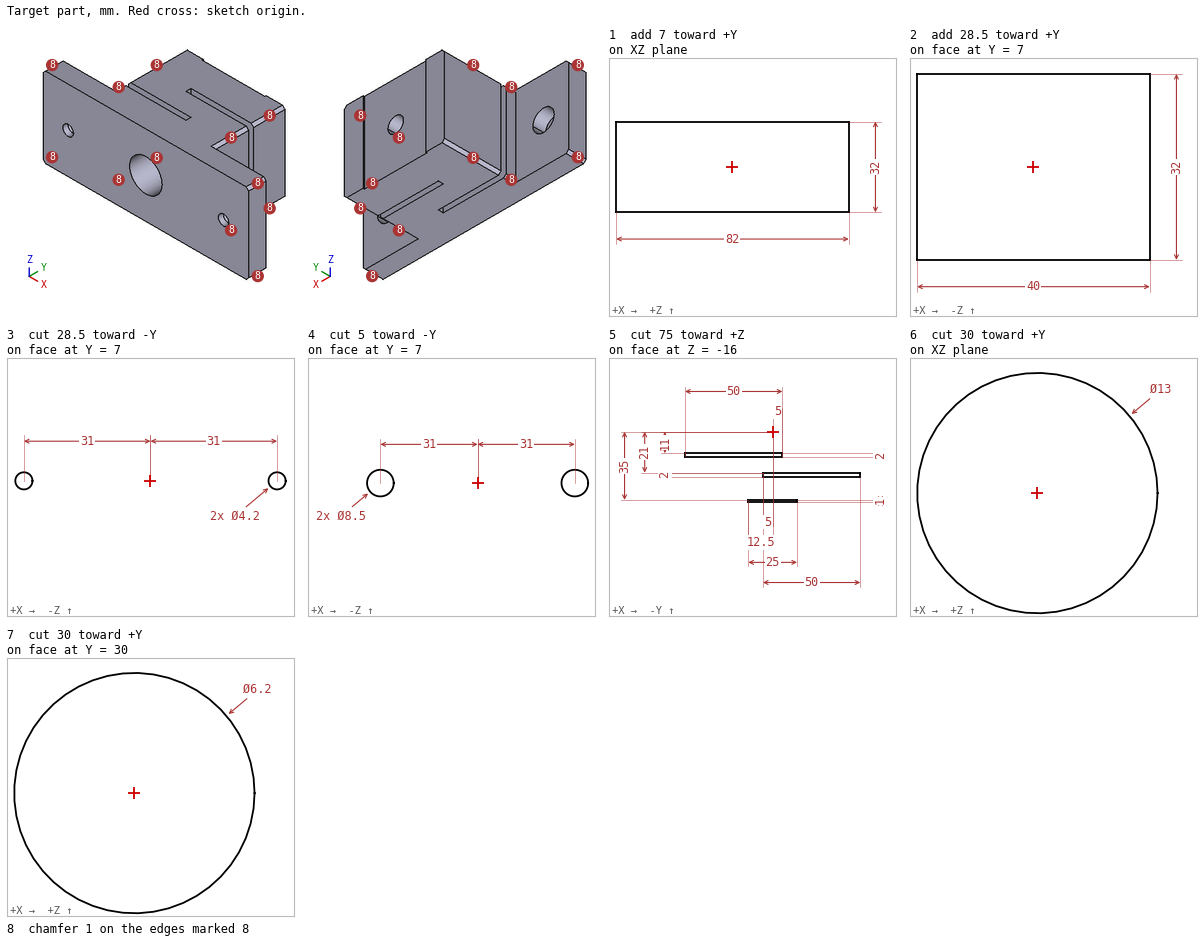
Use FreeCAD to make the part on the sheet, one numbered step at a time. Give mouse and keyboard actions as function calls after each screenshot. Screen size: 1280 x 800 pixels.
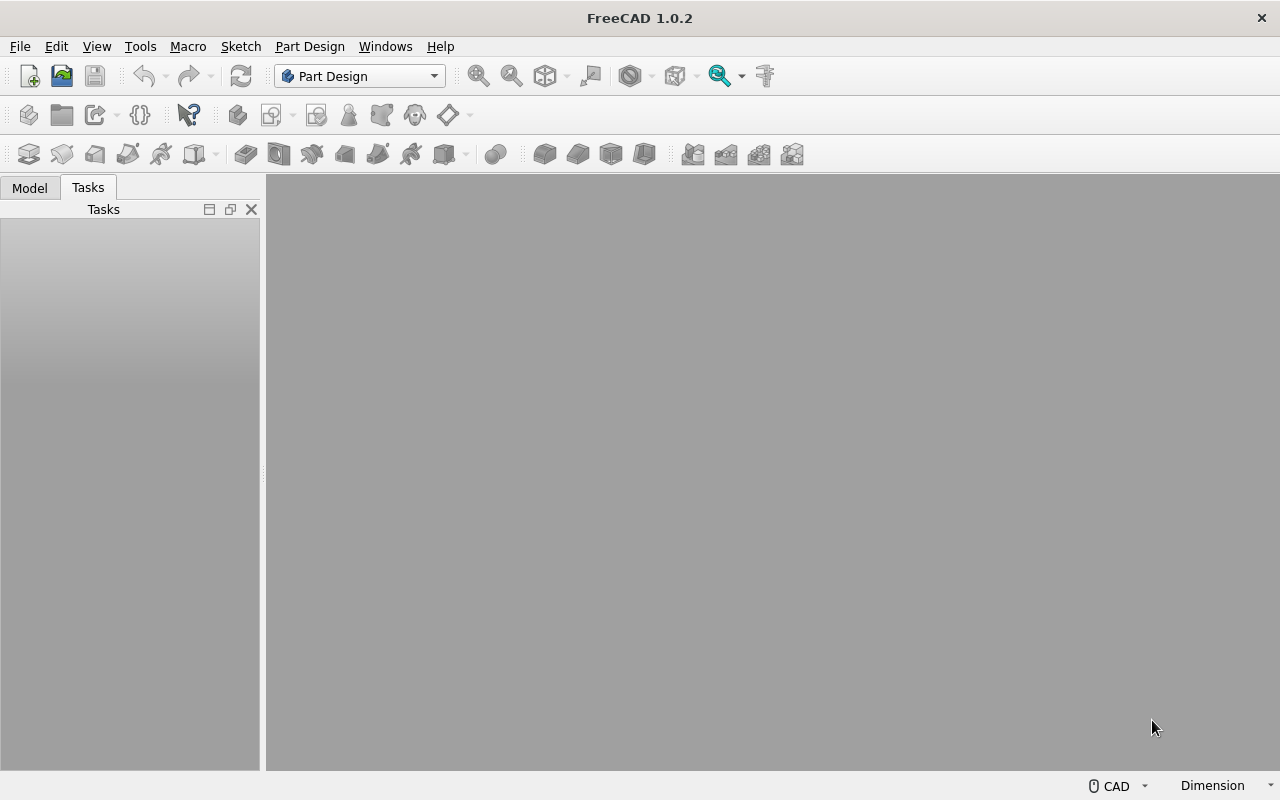
key(ctrl+n)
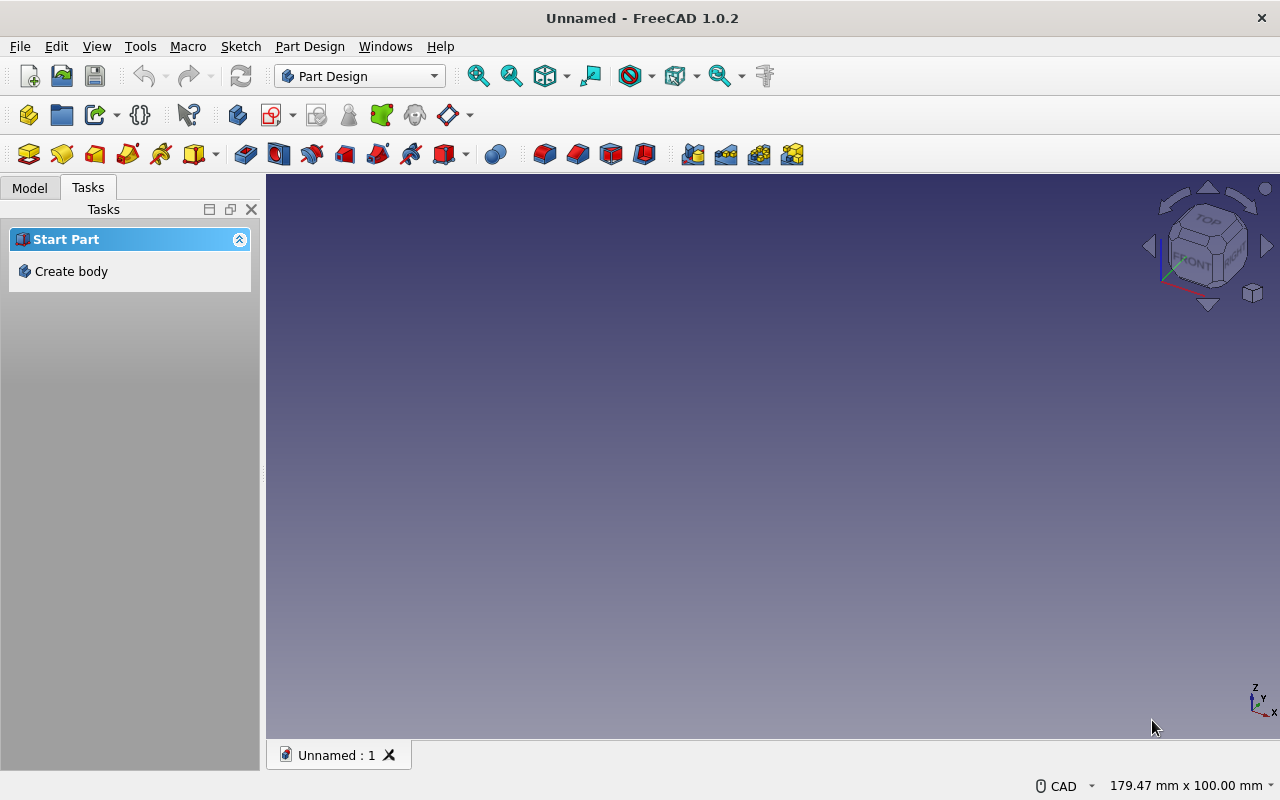
click(270, 116)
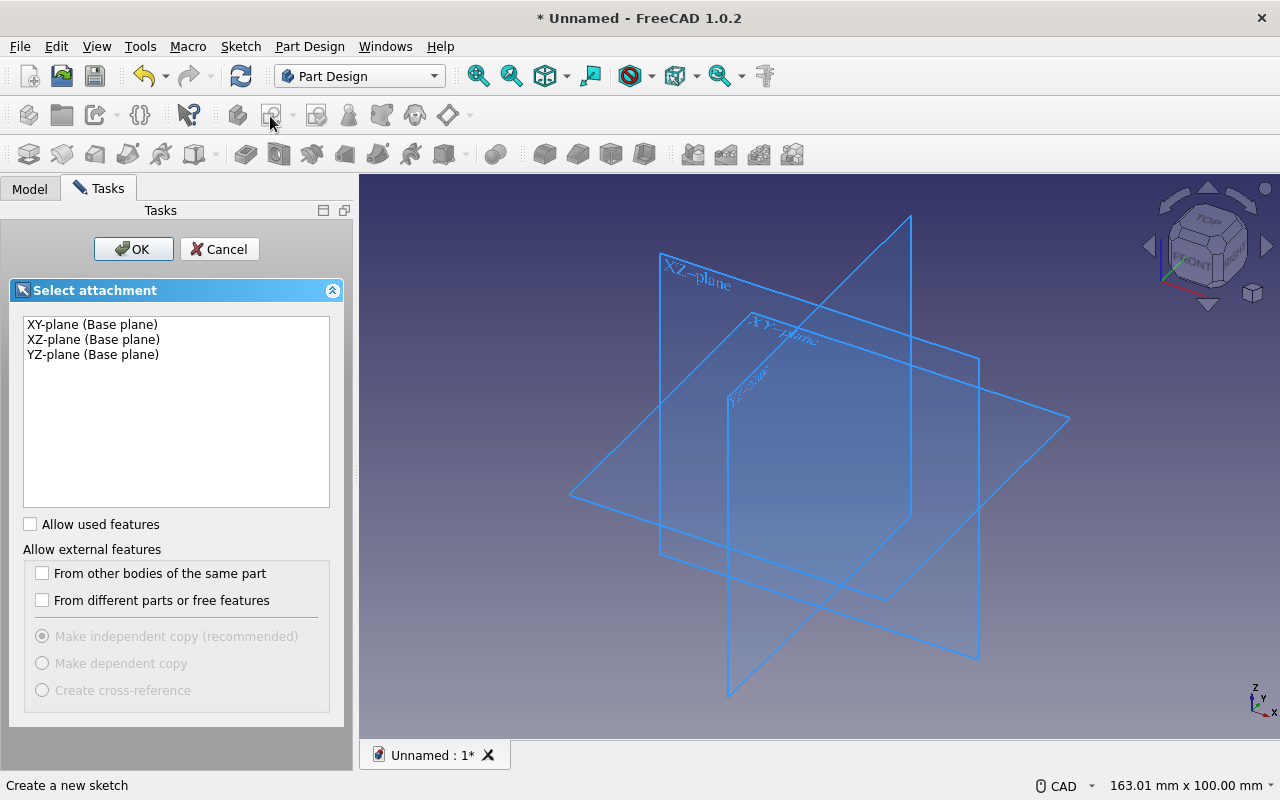
click(84, 340)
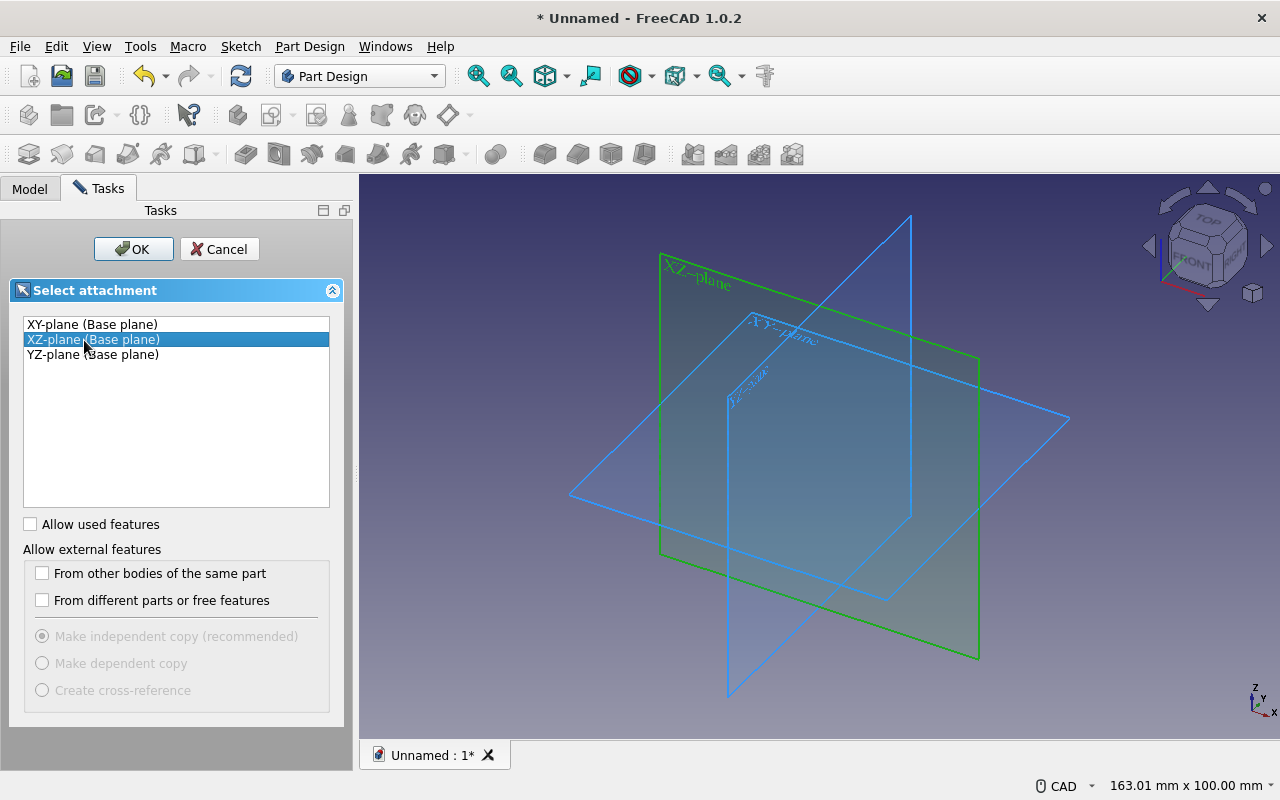
click(134, 249)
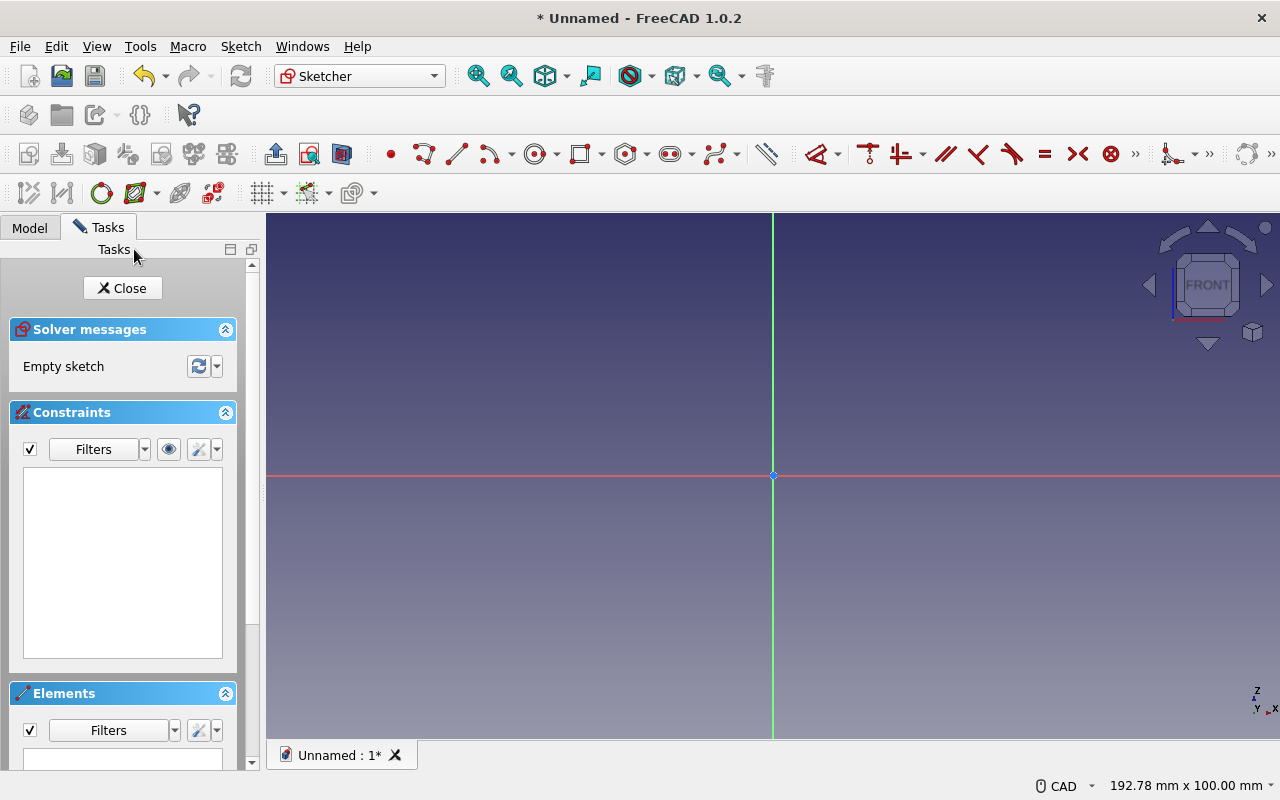
key(g)
key(v)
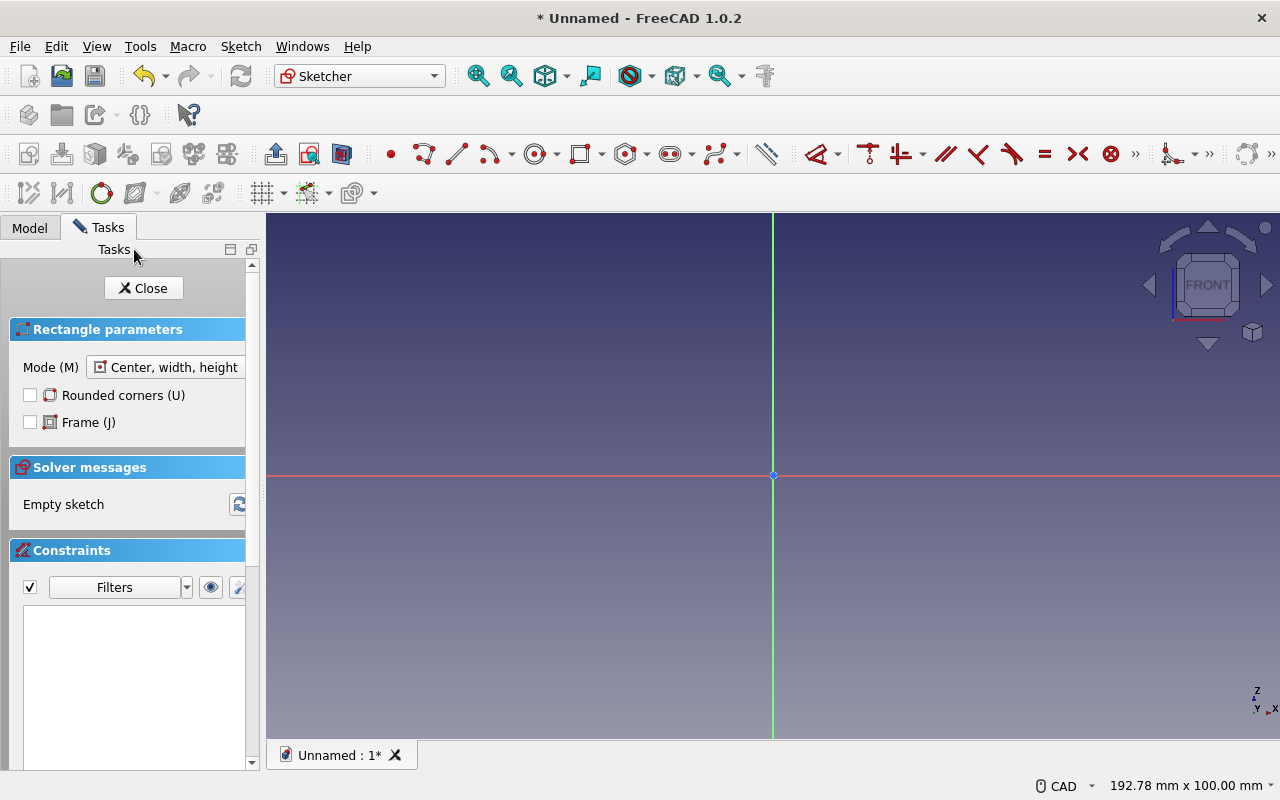
click(773, 476)
move(989, 392)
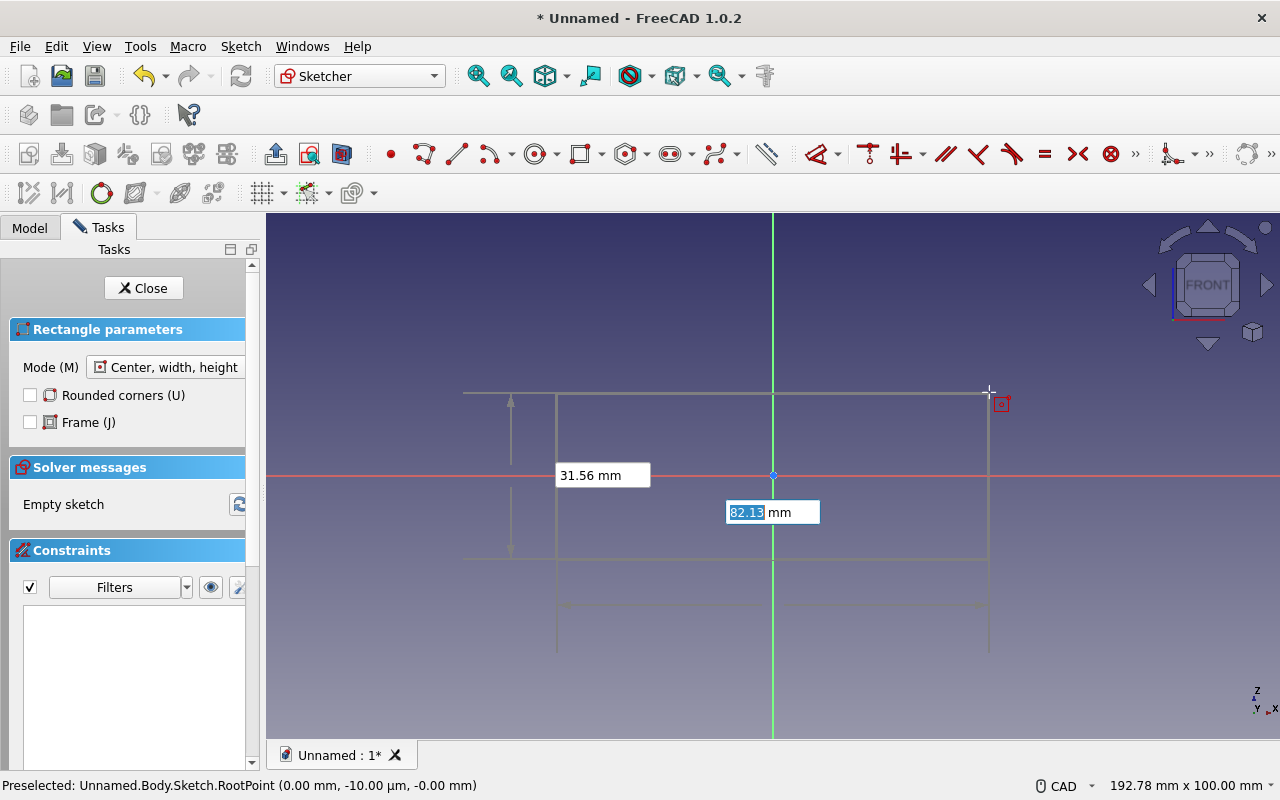
text(82)
key(Tab)
text(32)
key(Return)
key(Escape)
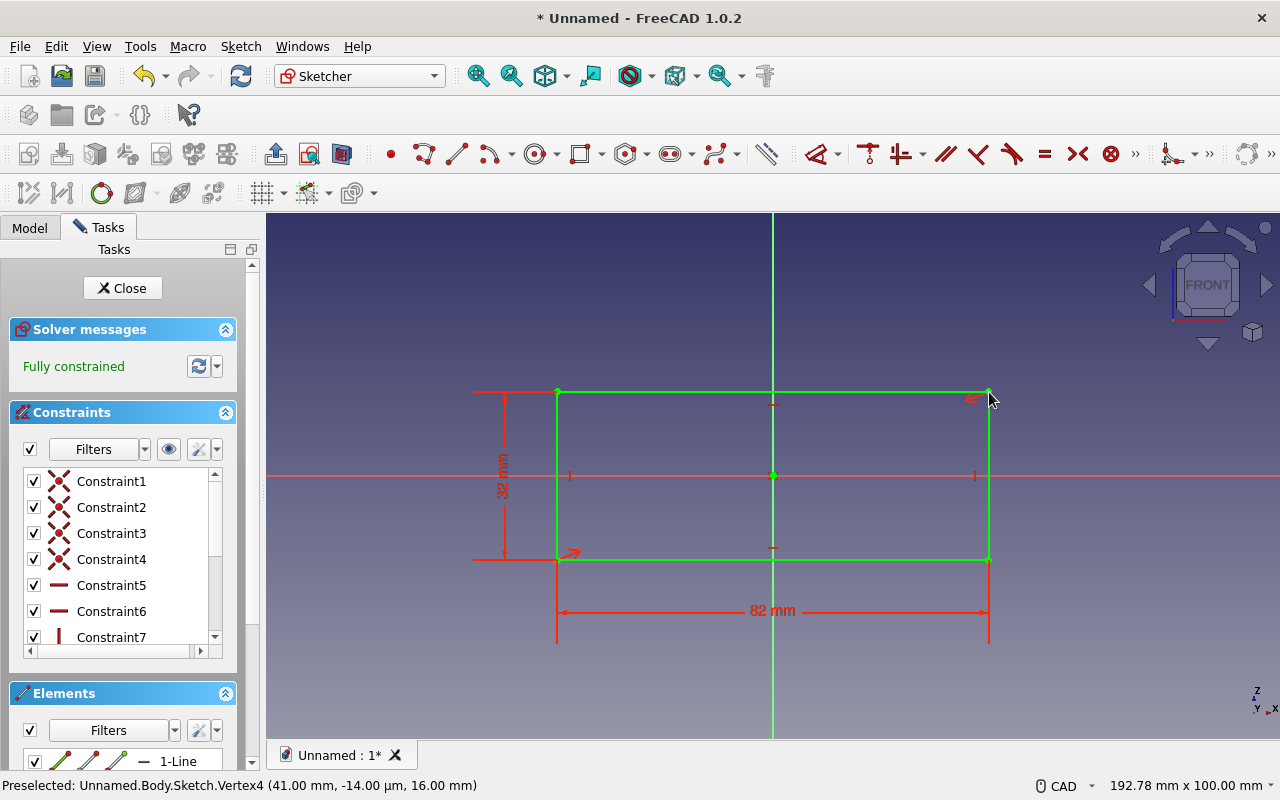
click(123, 288)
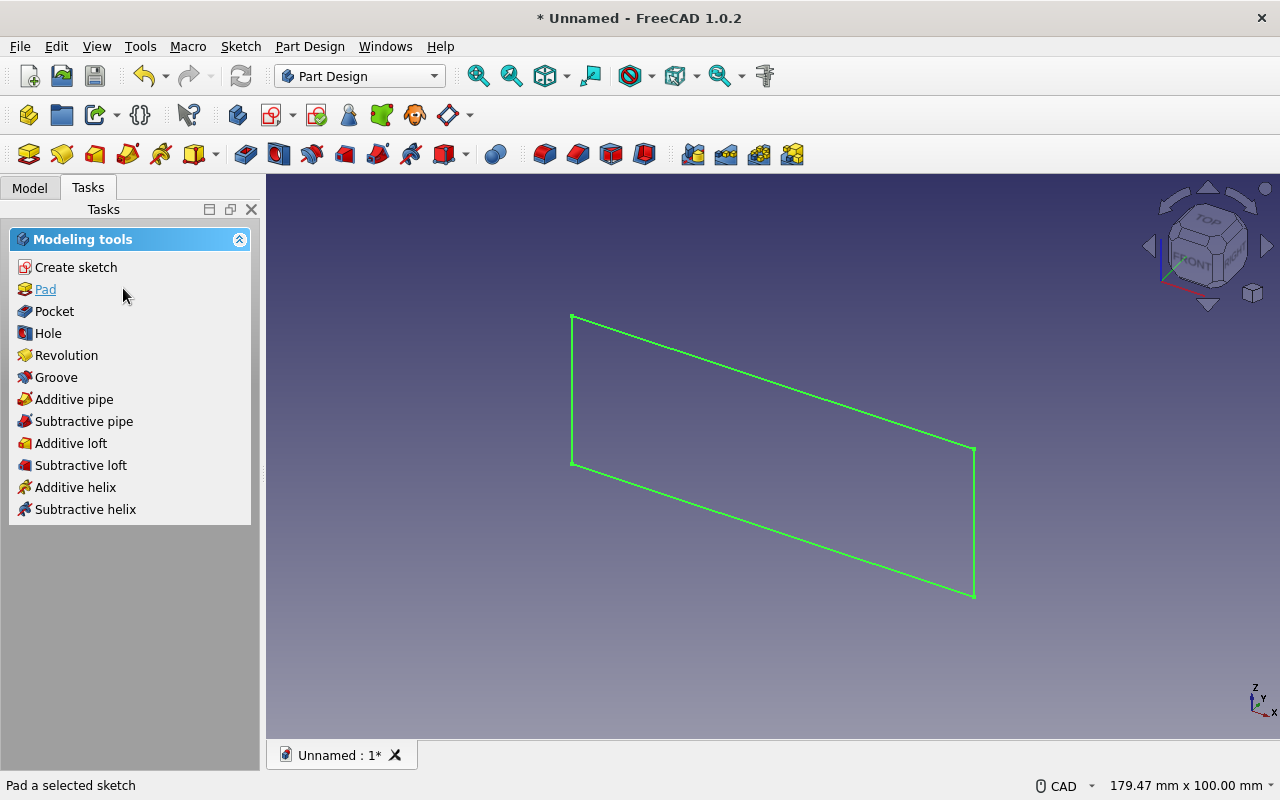
click(29, 154)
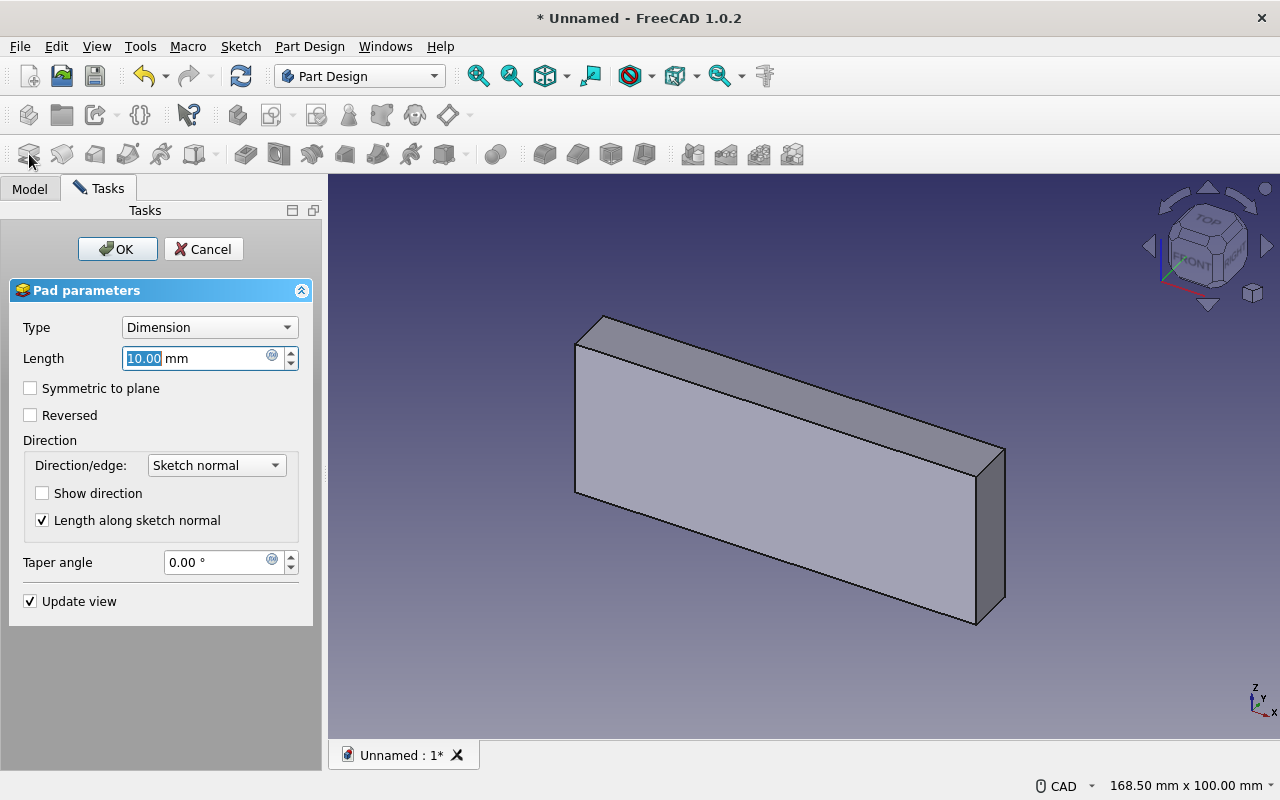
text(7)
key(Tab)